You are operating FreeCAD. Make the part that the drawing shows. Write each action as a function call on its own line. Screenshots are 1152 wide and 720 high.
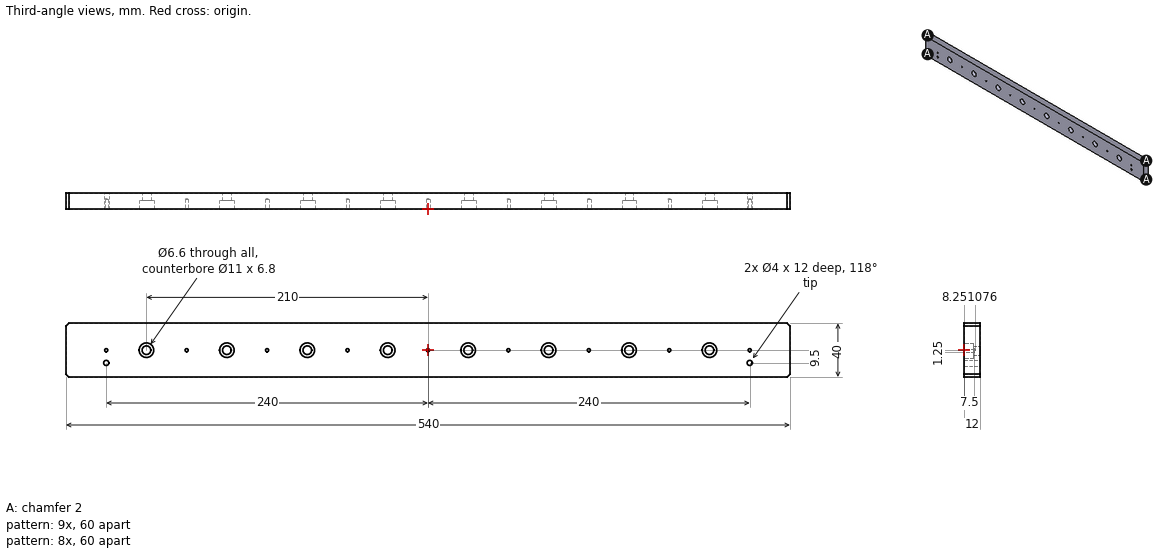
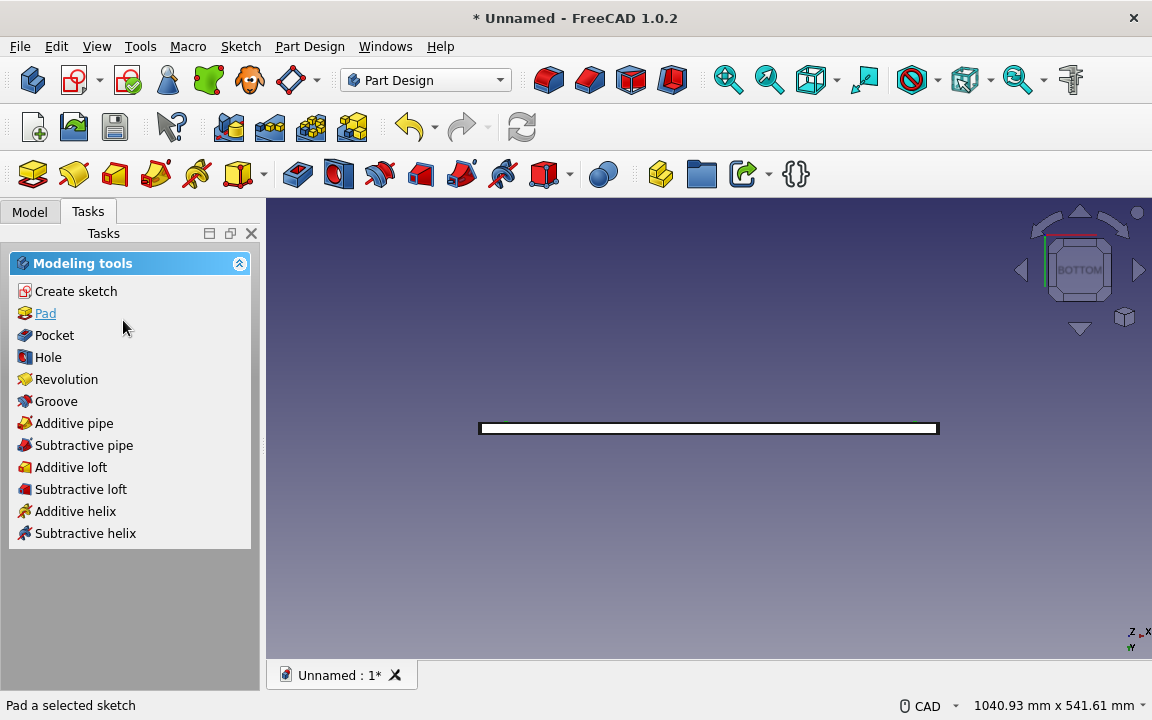
click(339, 174)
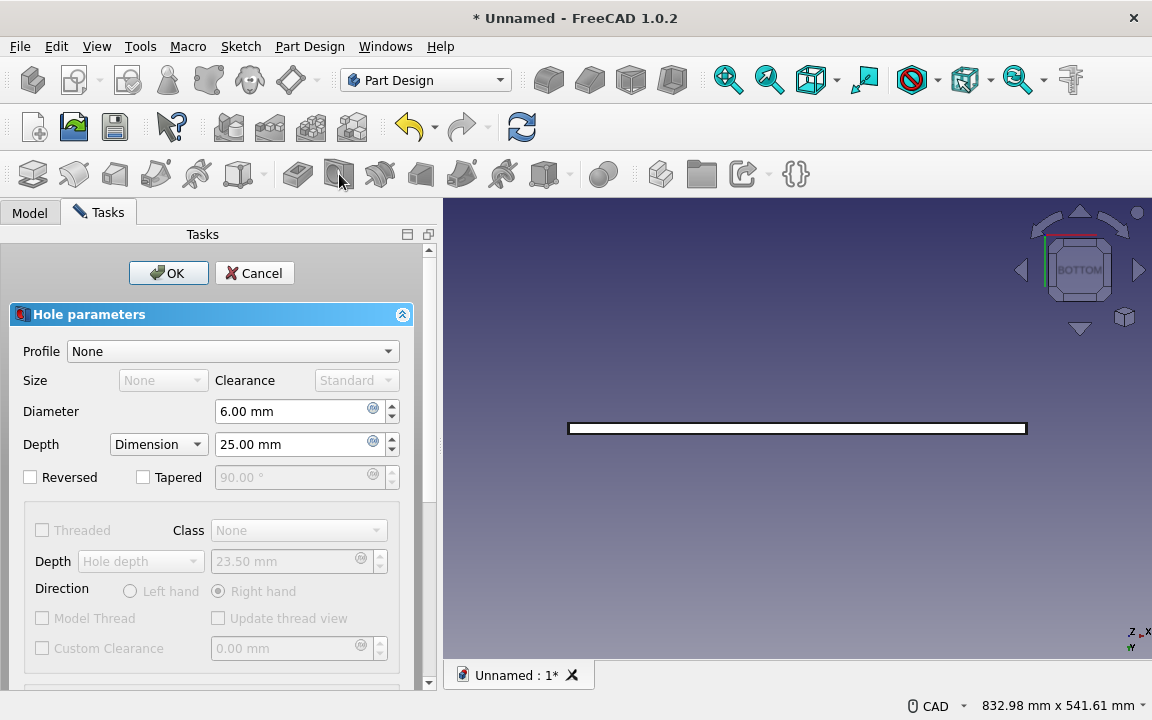
triple_click(300, 412)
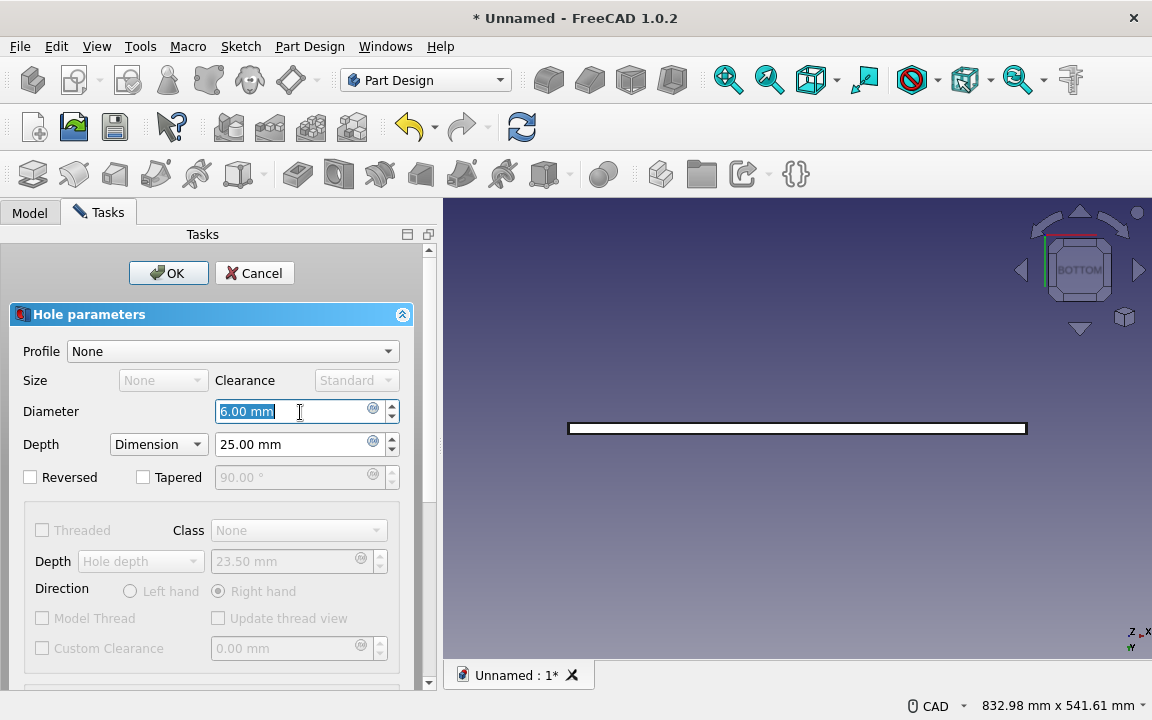
text(4)
key(Tab)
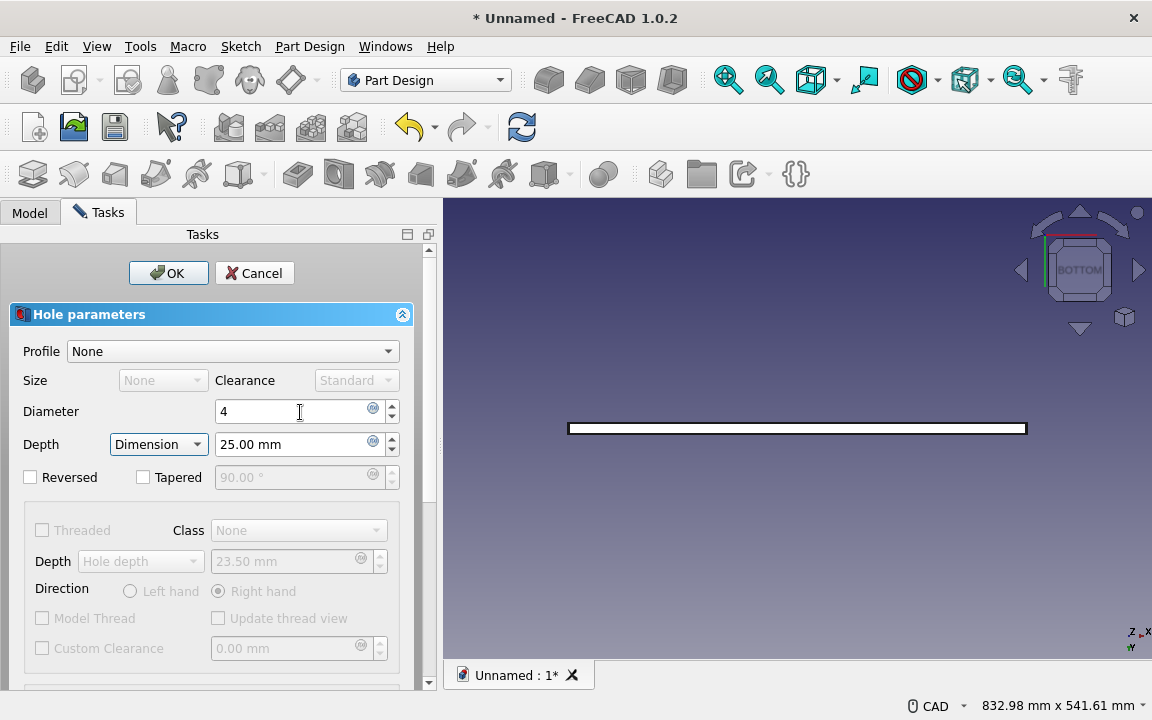
triple_click(300, 444)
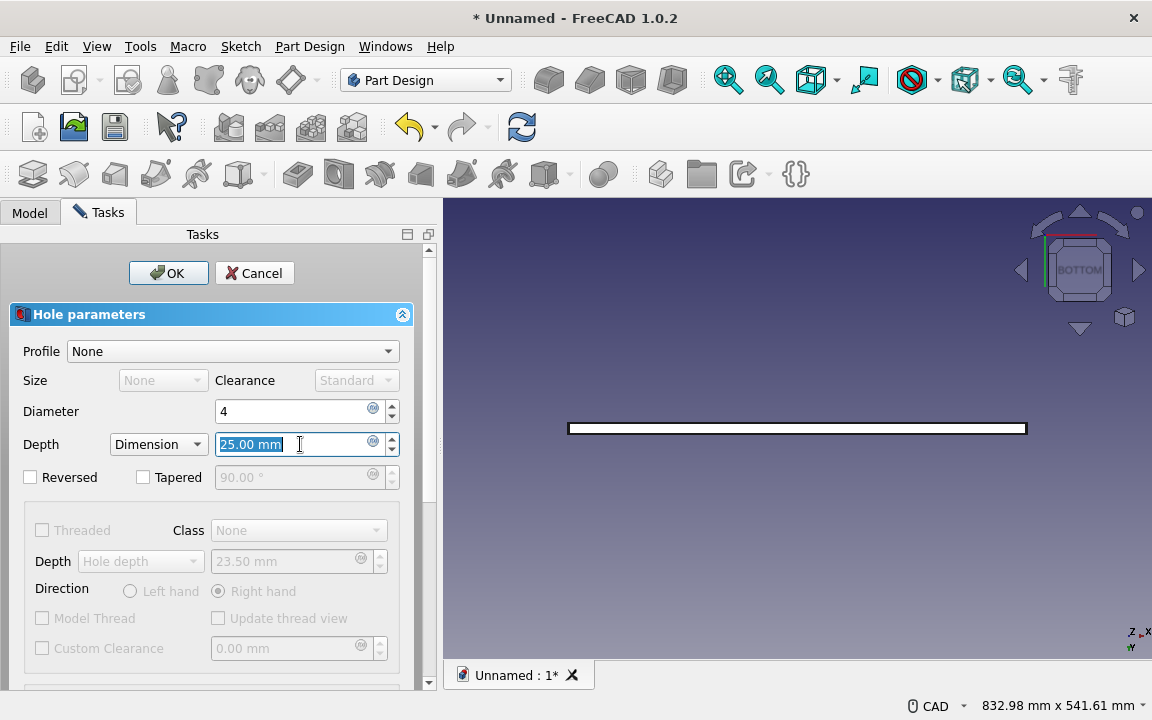
text(12)
key(Tab)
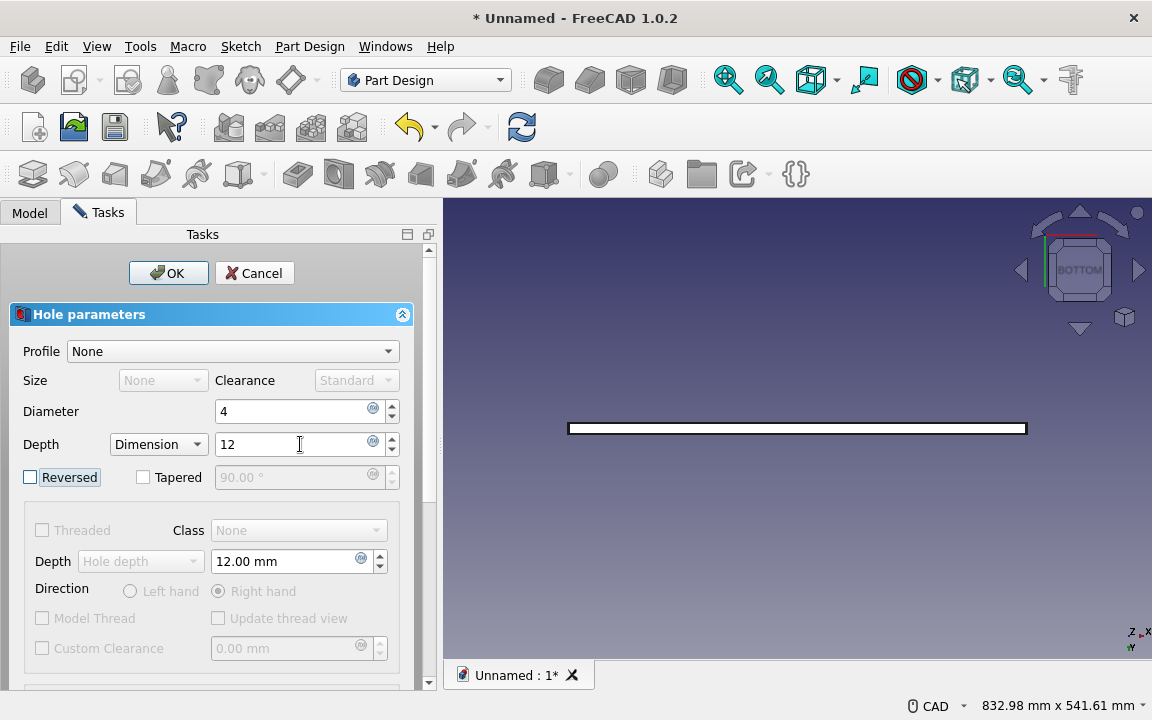
click(169, 273)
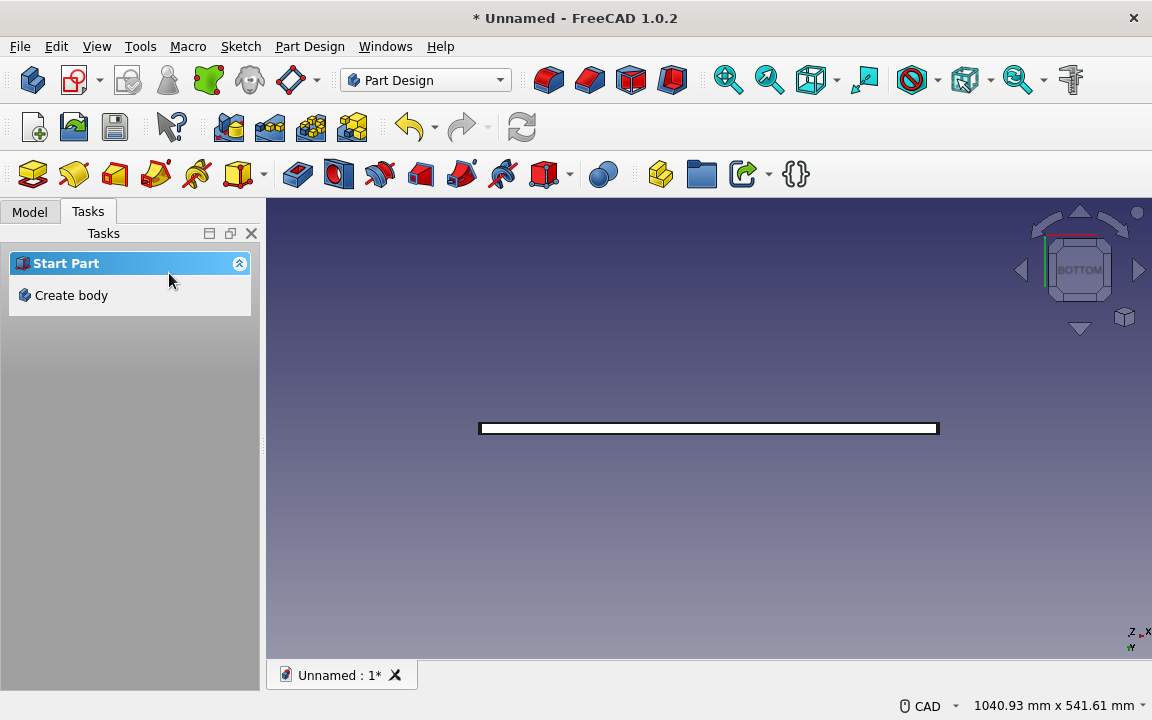
click(30, 212)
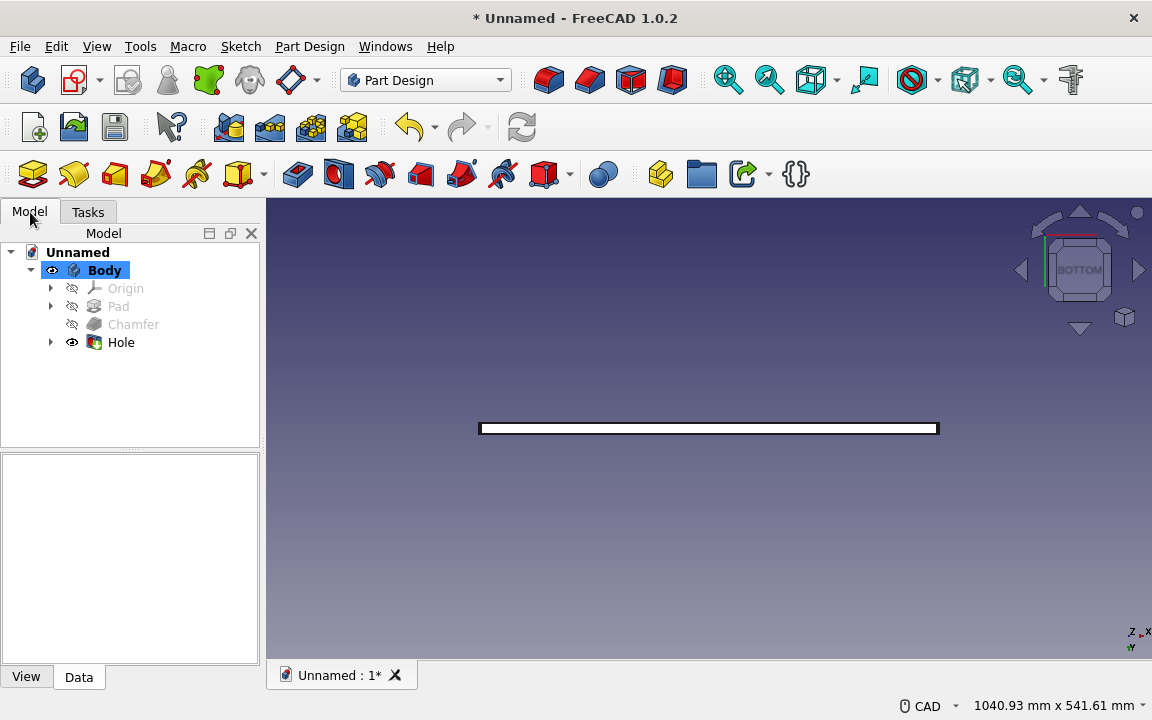
click(51, 288)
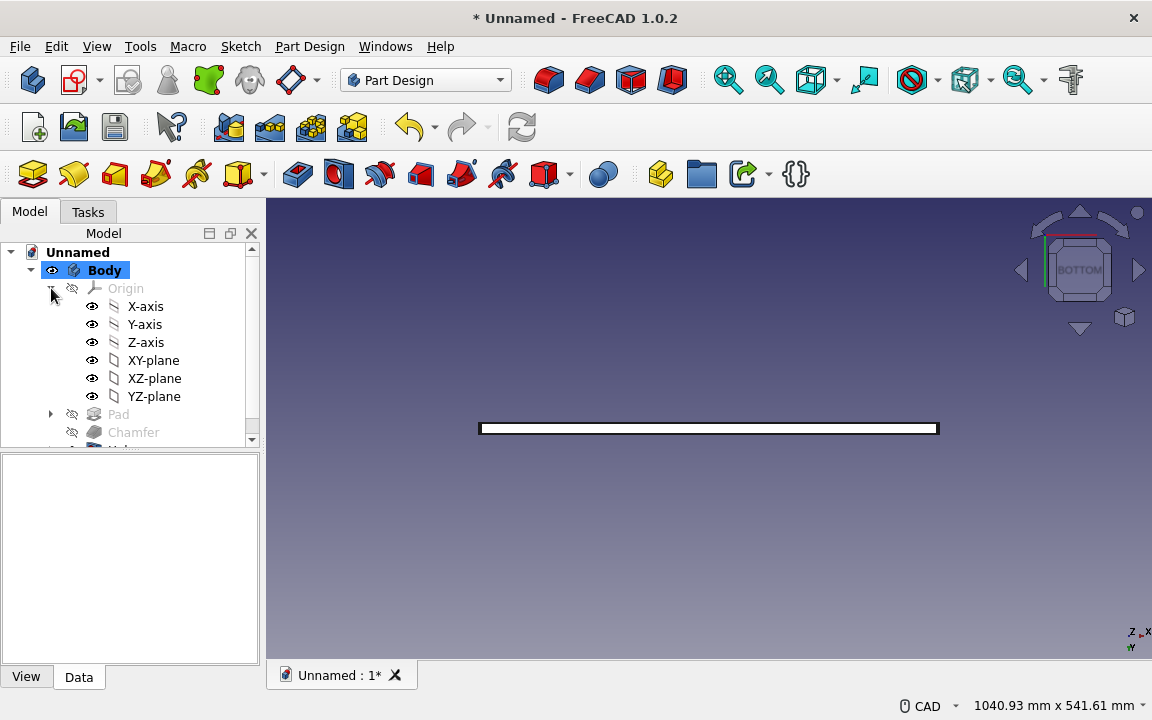
click(137, 396)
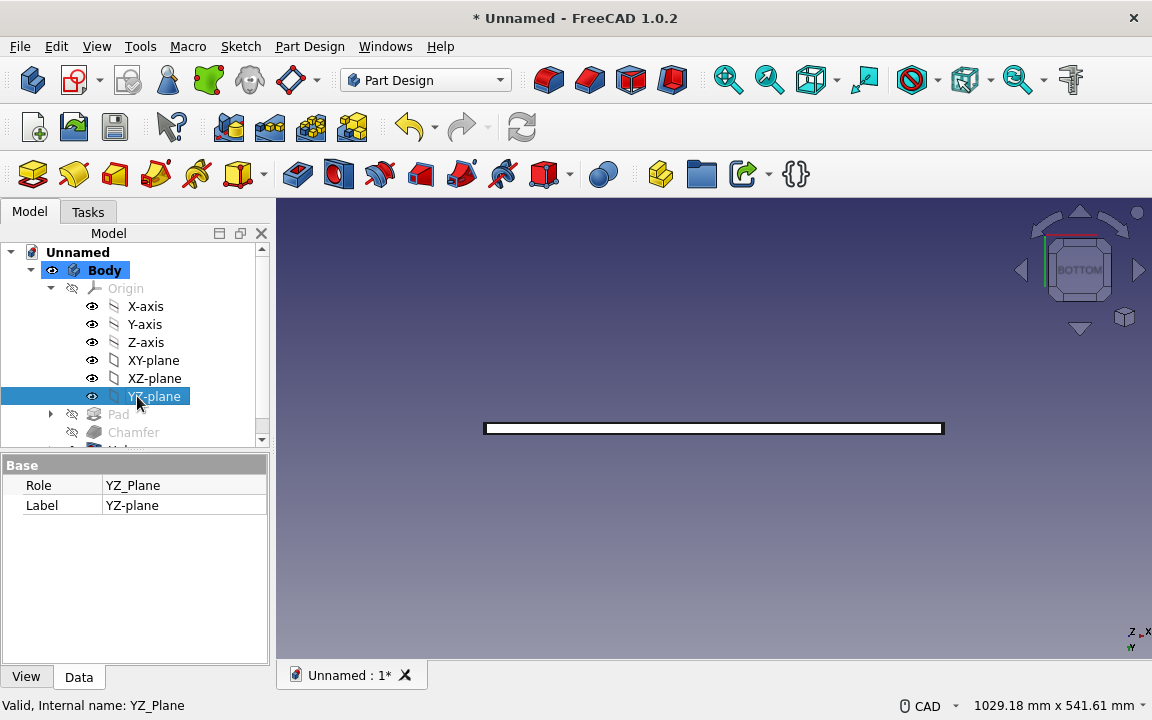
click(290, 80)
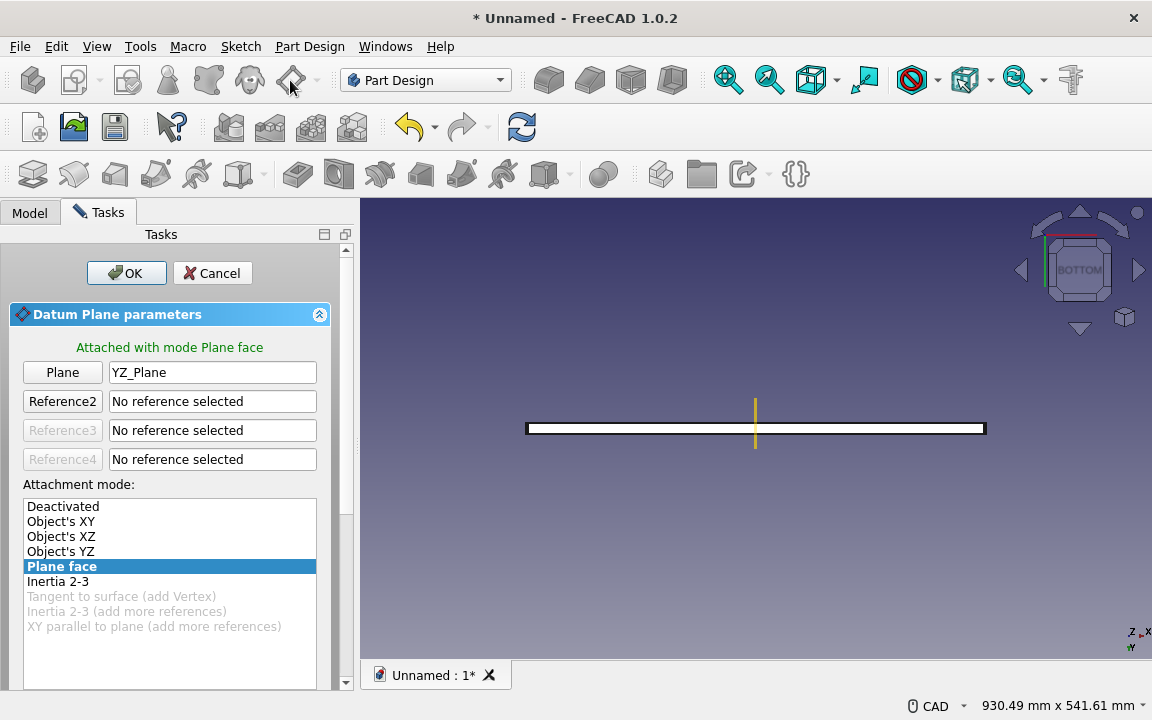
scroll(346, 467, down, 4)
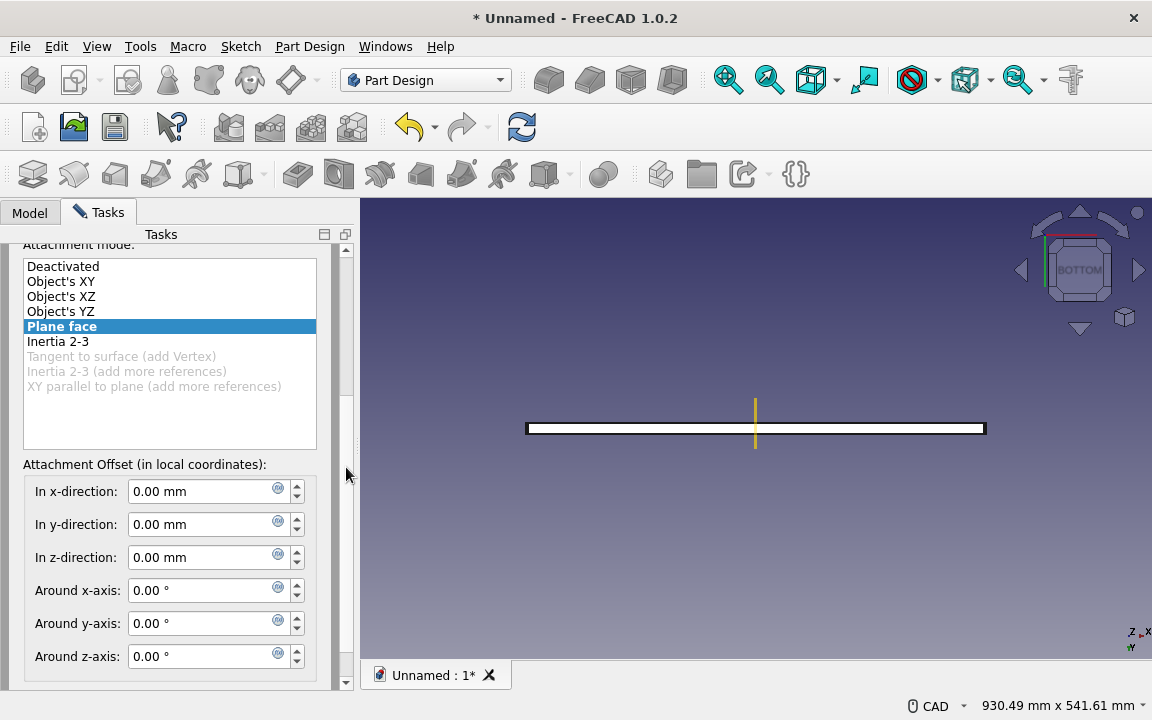
triple_click(210, 558)